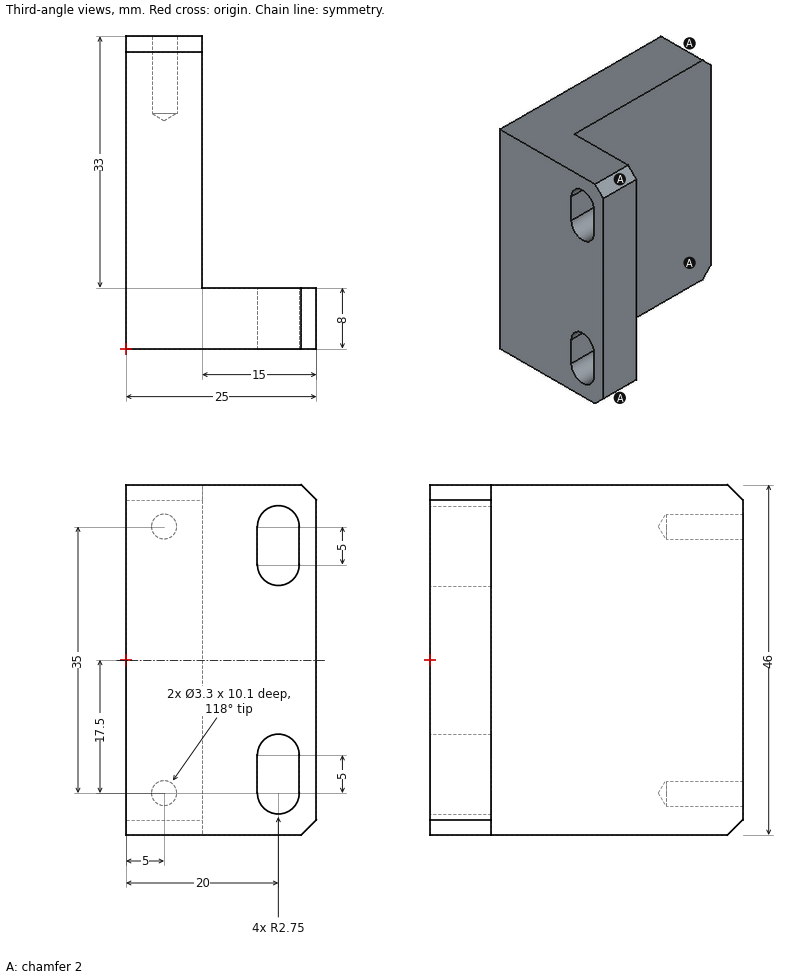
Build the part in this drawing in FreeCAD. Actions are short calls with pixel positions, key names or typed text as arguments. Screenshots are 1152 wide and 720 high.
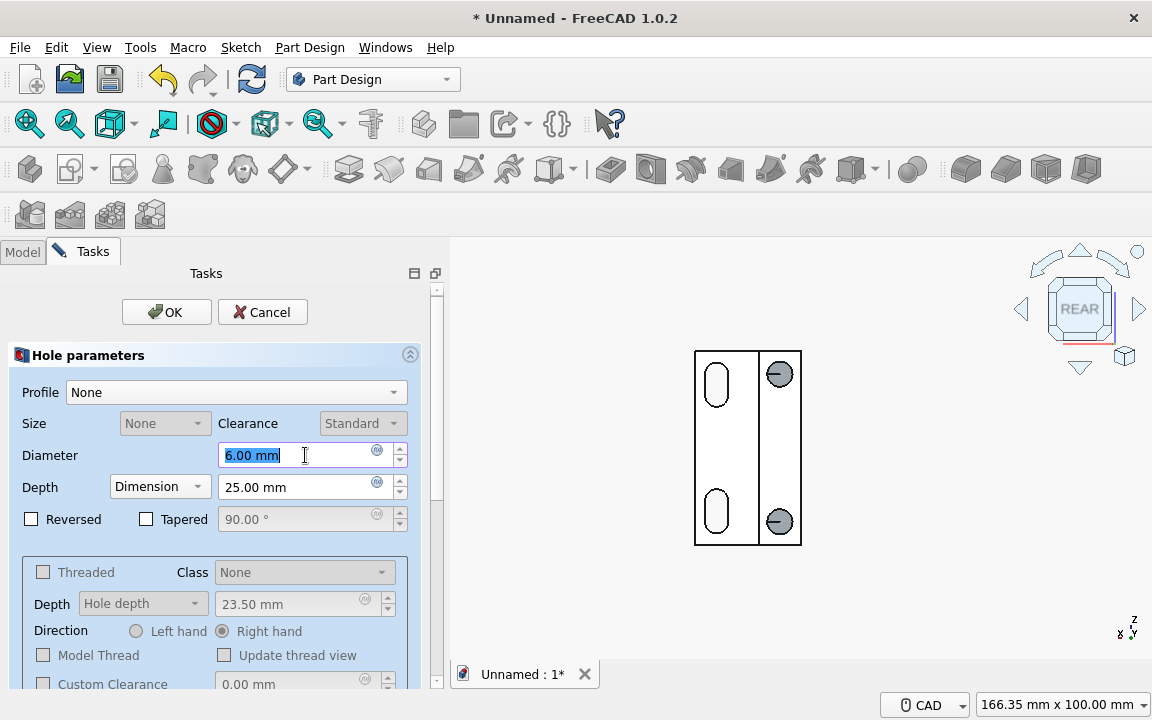
text(3.3)
key(Tab)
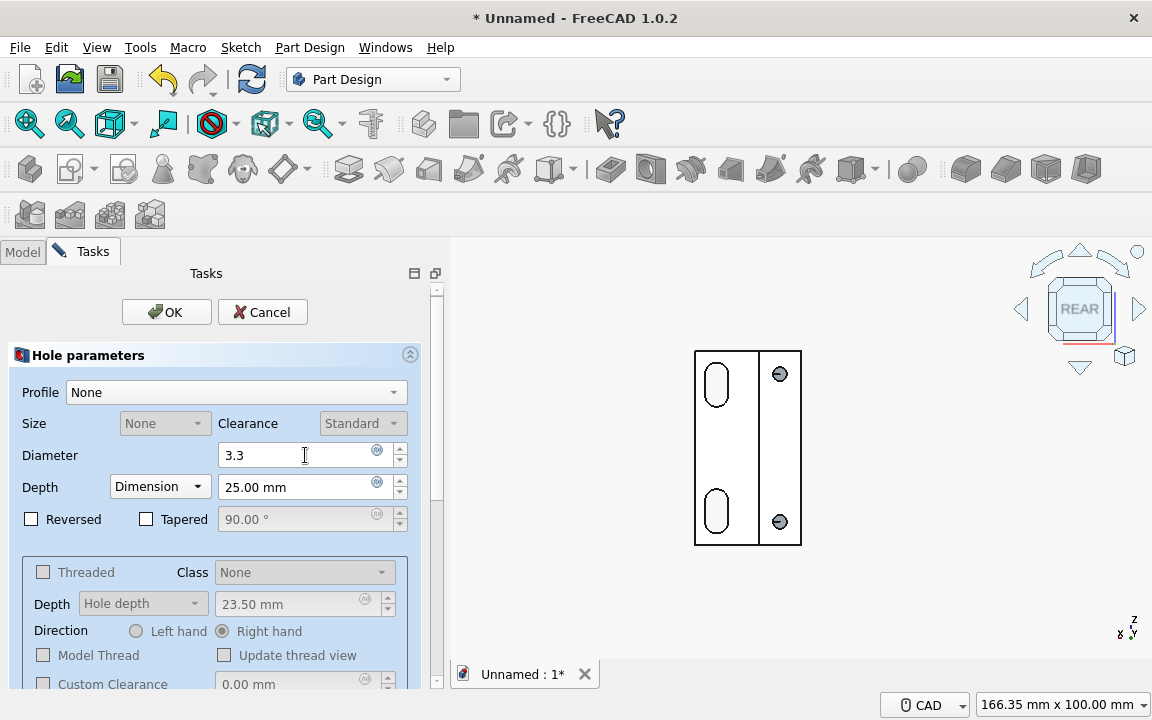
triple_click(305, 487)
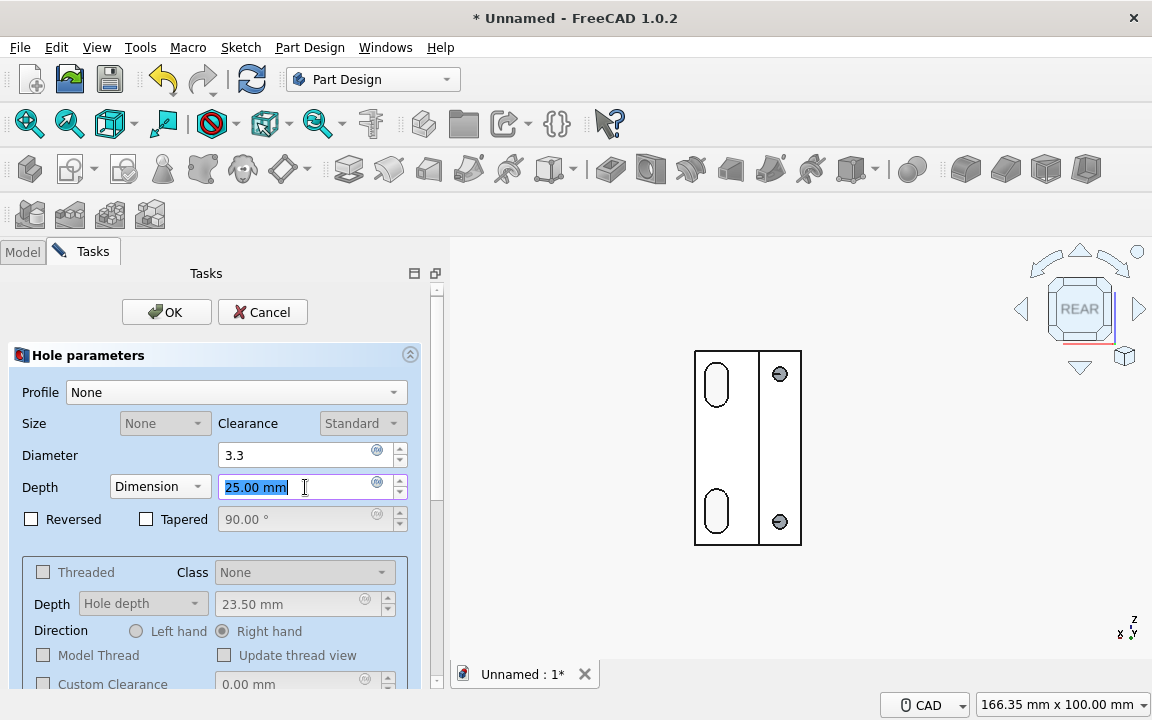
text(10.1)
key(Tab)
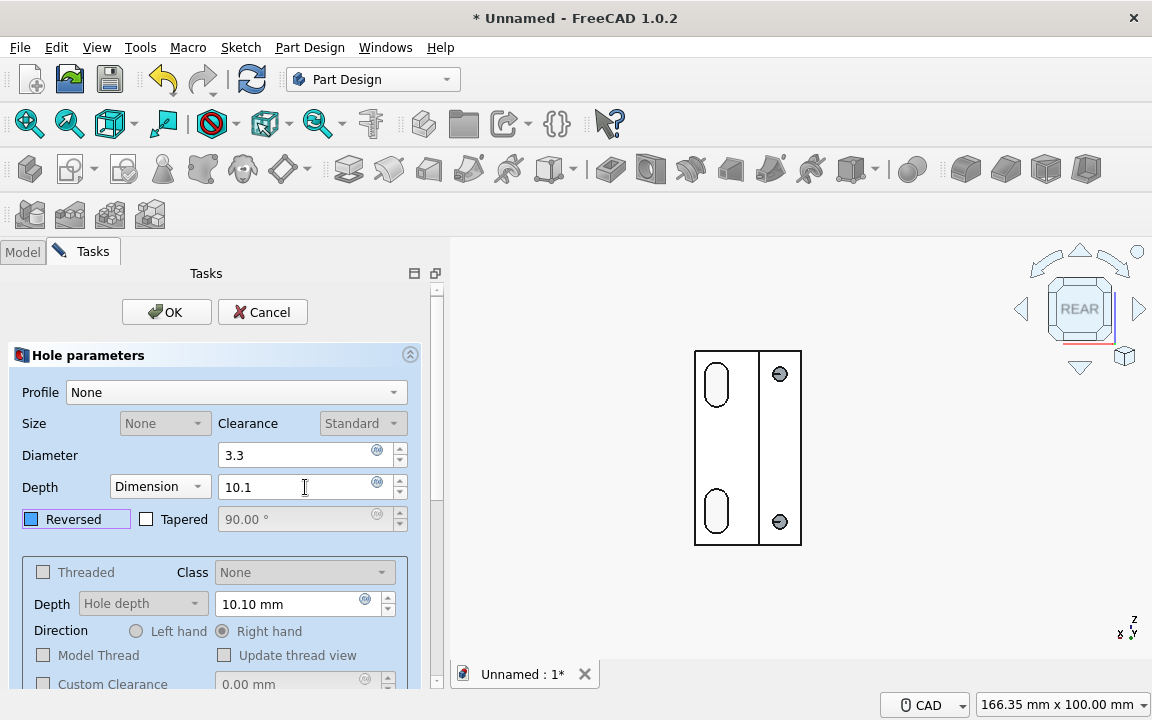
click(167, 312)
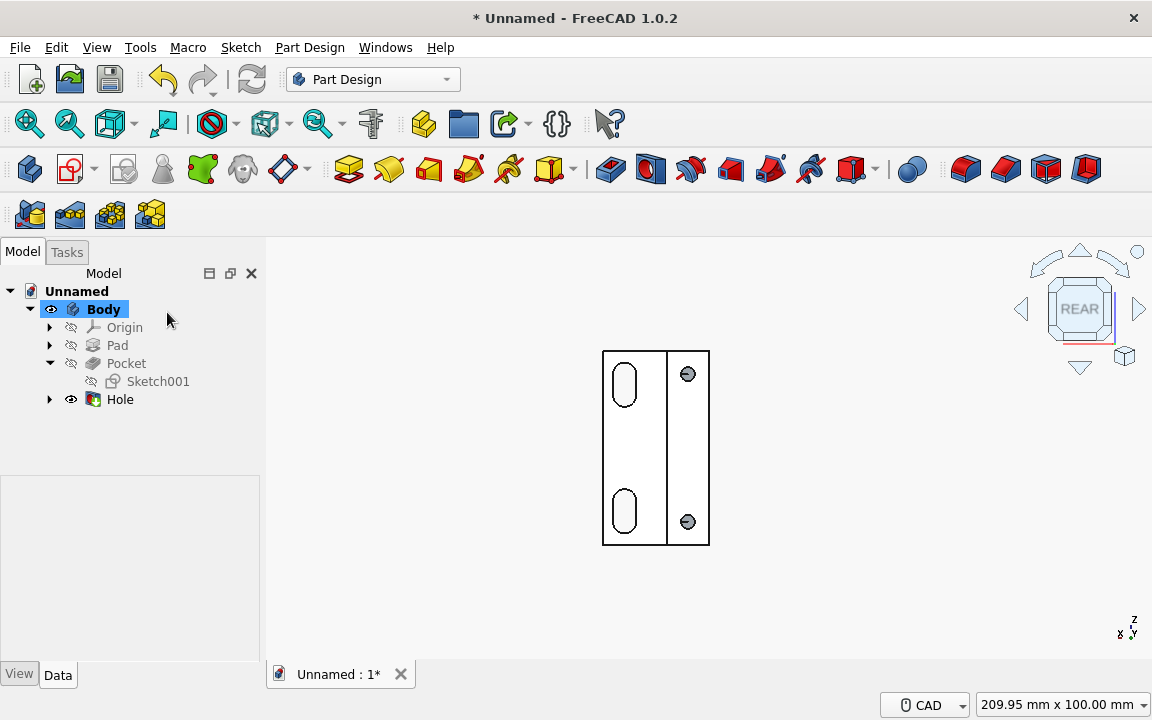
click(688, 350)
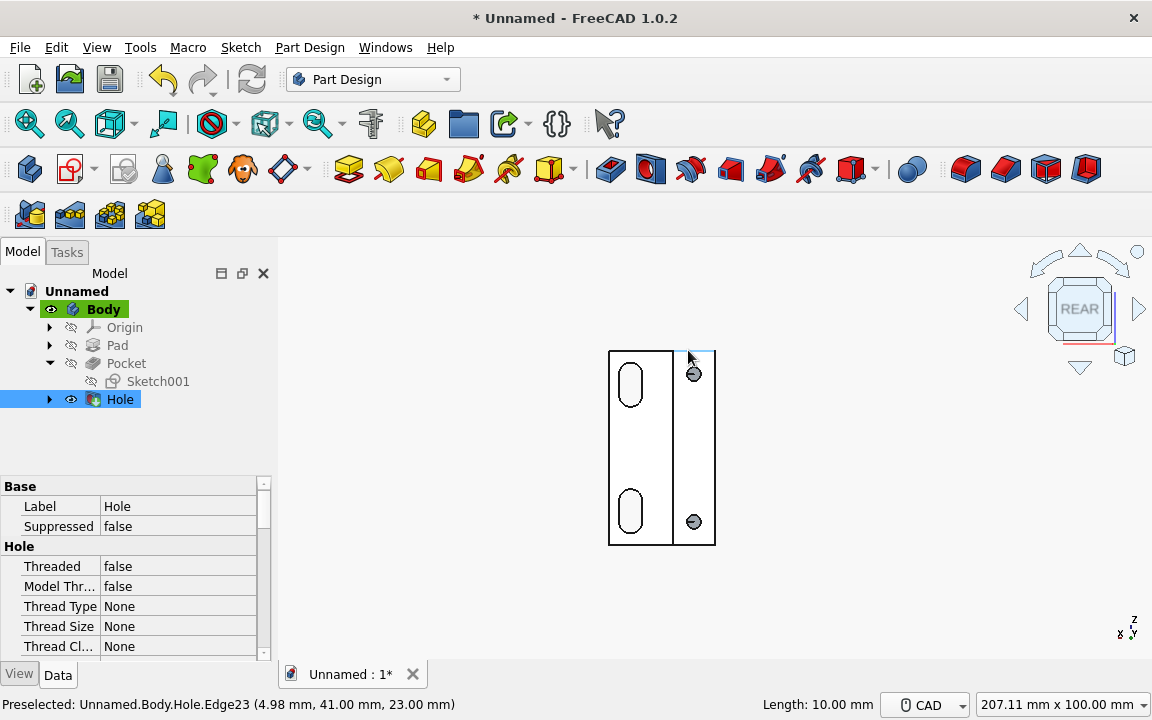
click(694, 544, ctrl)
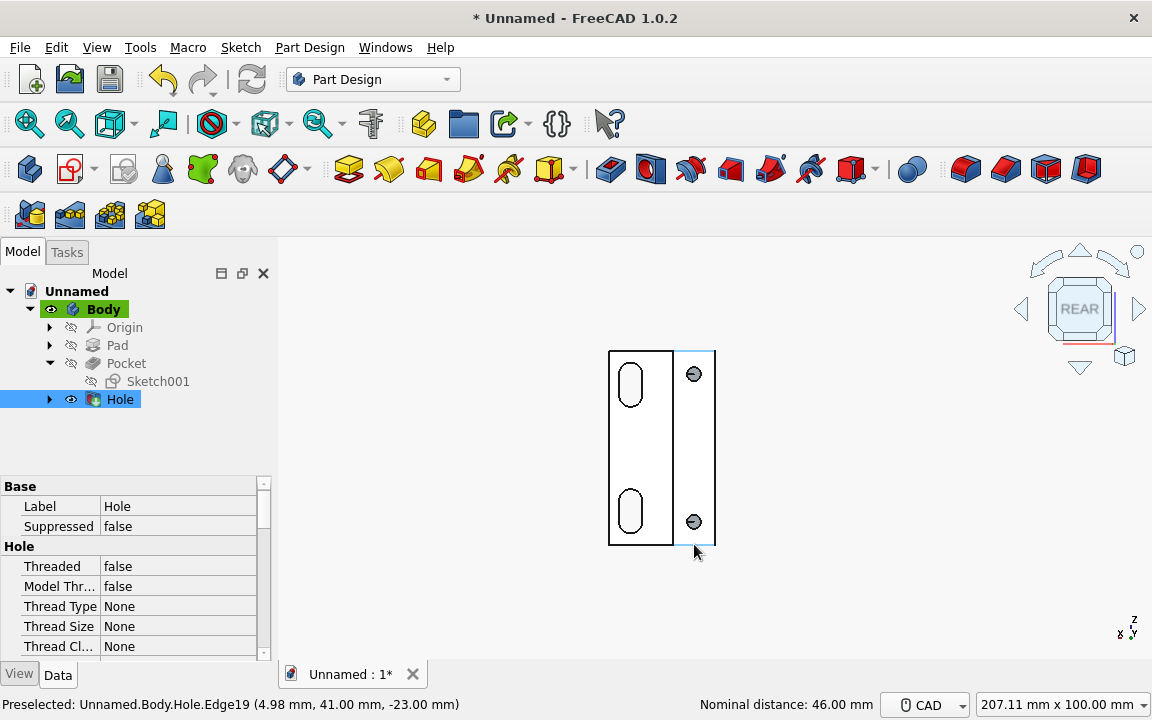
key(0)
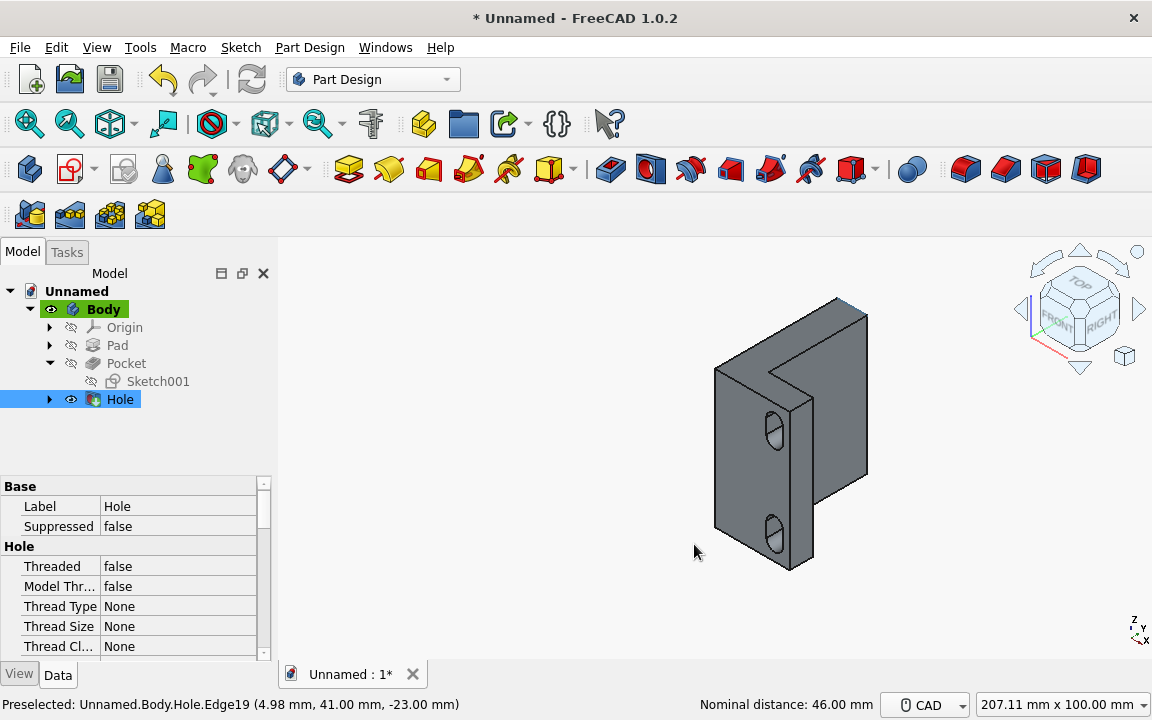
click(802, 404, ctrl)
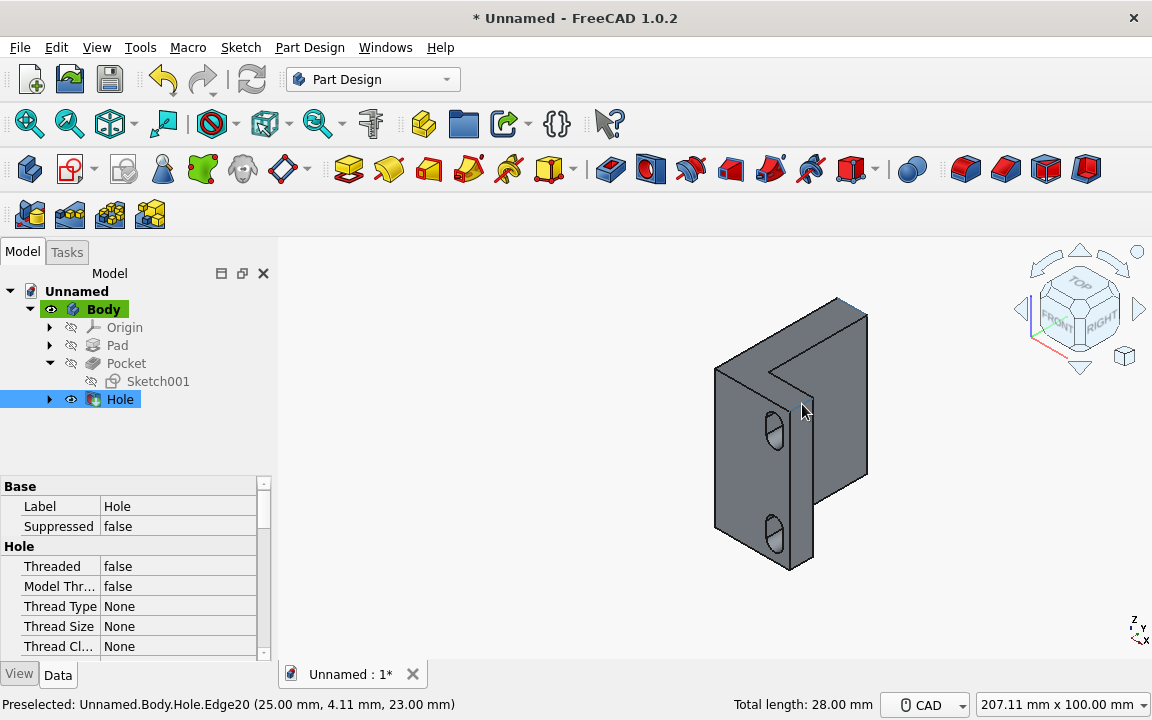
key(2)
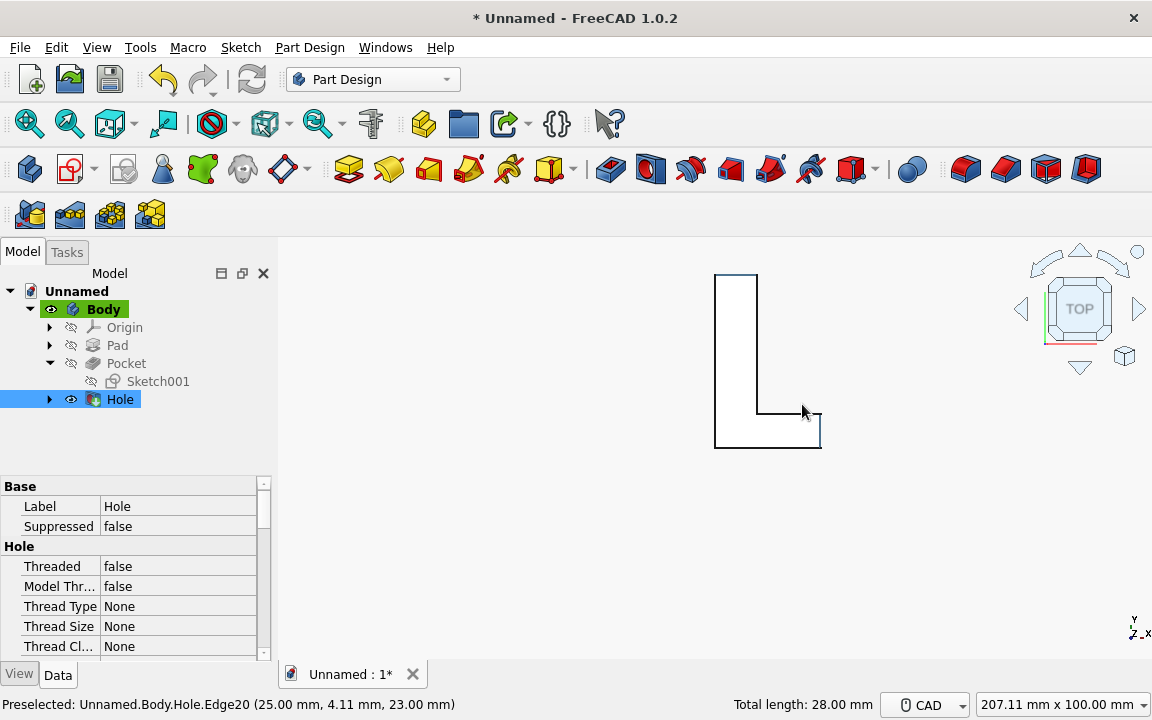
key(v)
key(f)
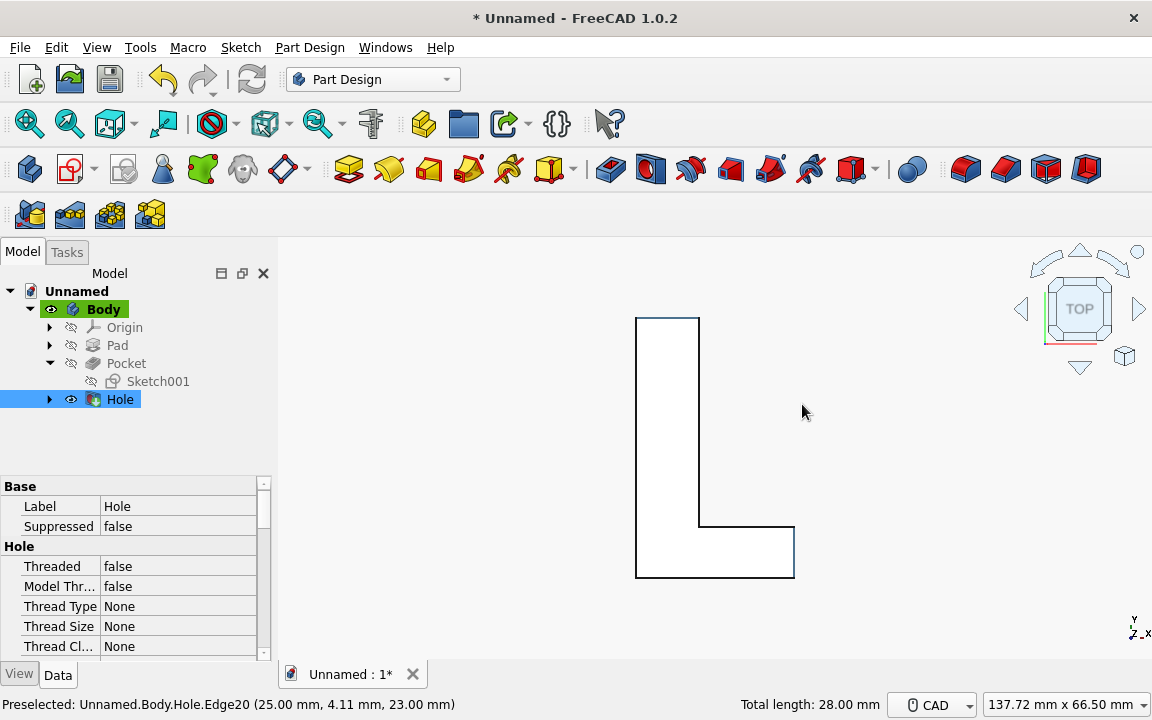
key(1)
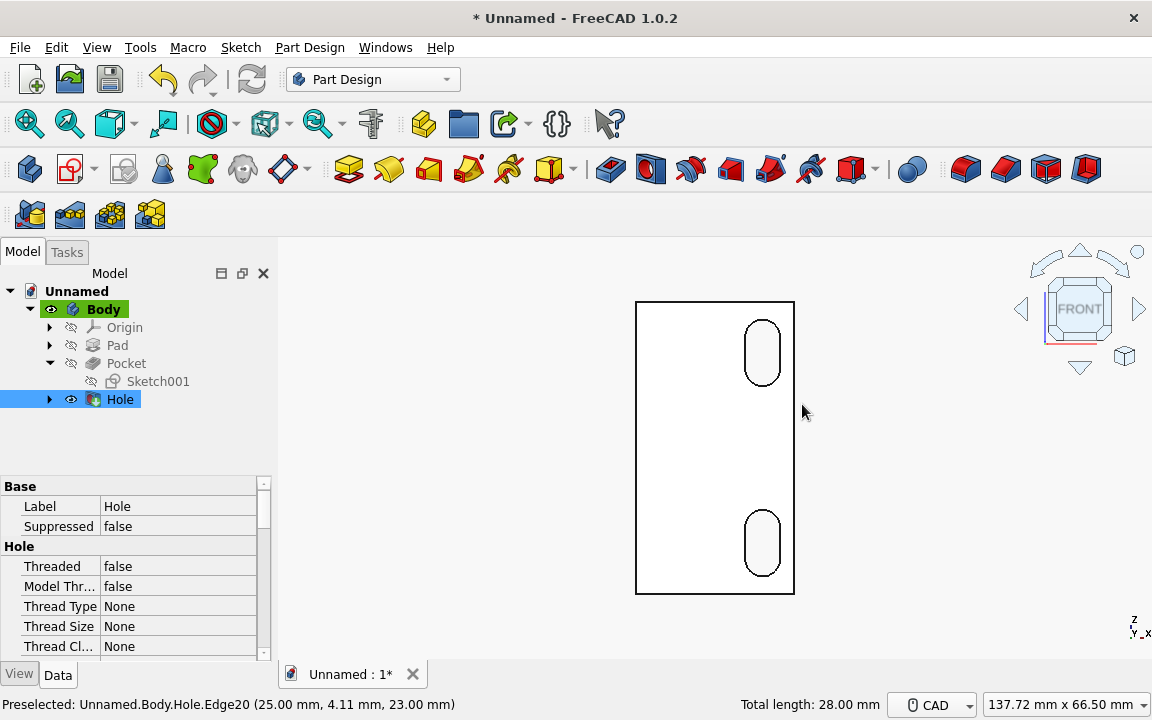
key(3)